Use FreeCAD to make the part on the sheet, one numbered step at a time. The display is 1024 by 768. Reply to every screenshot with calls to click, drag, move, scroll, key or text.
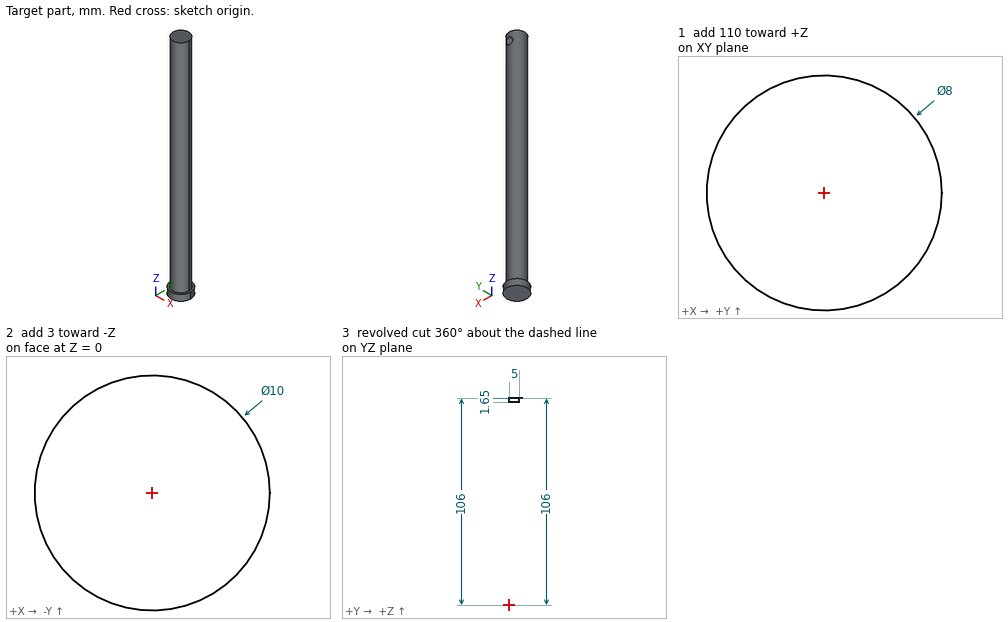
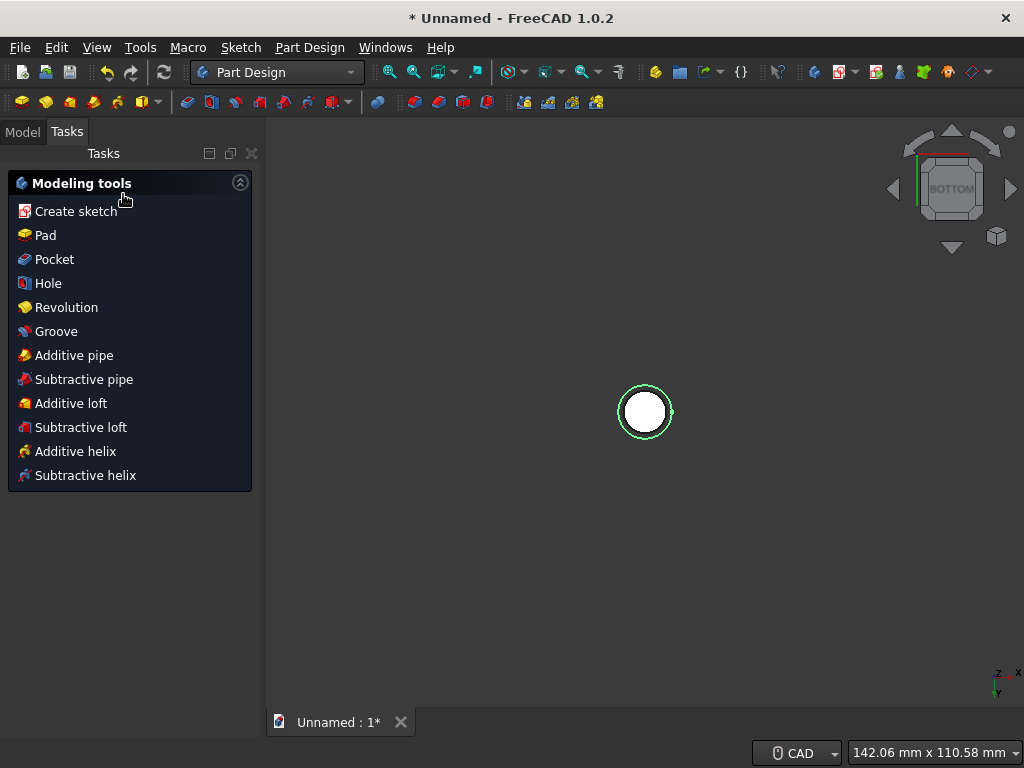
click(22, 102)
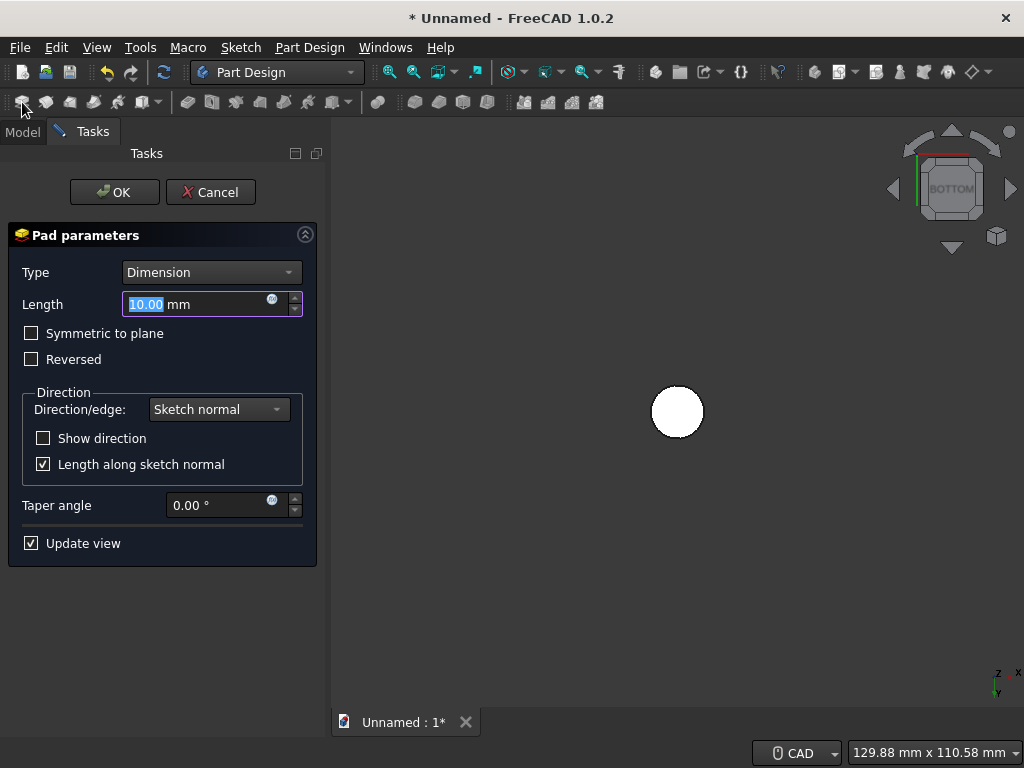
text(3)
key(Tab)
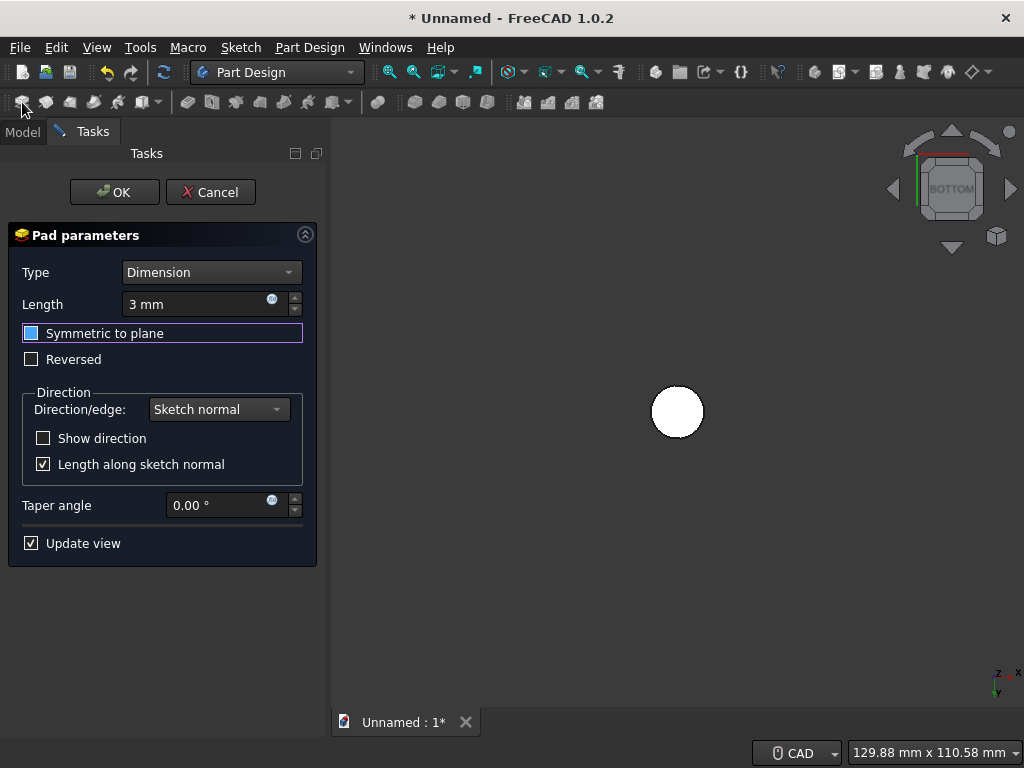
click(115, 192)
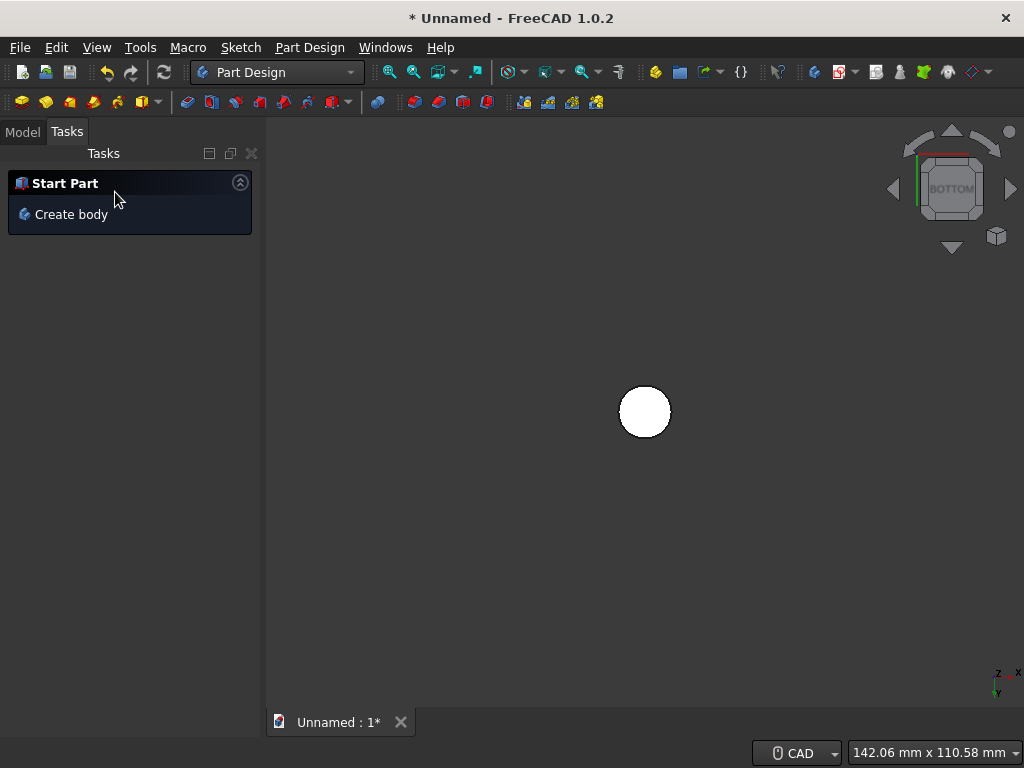
click(390, 72)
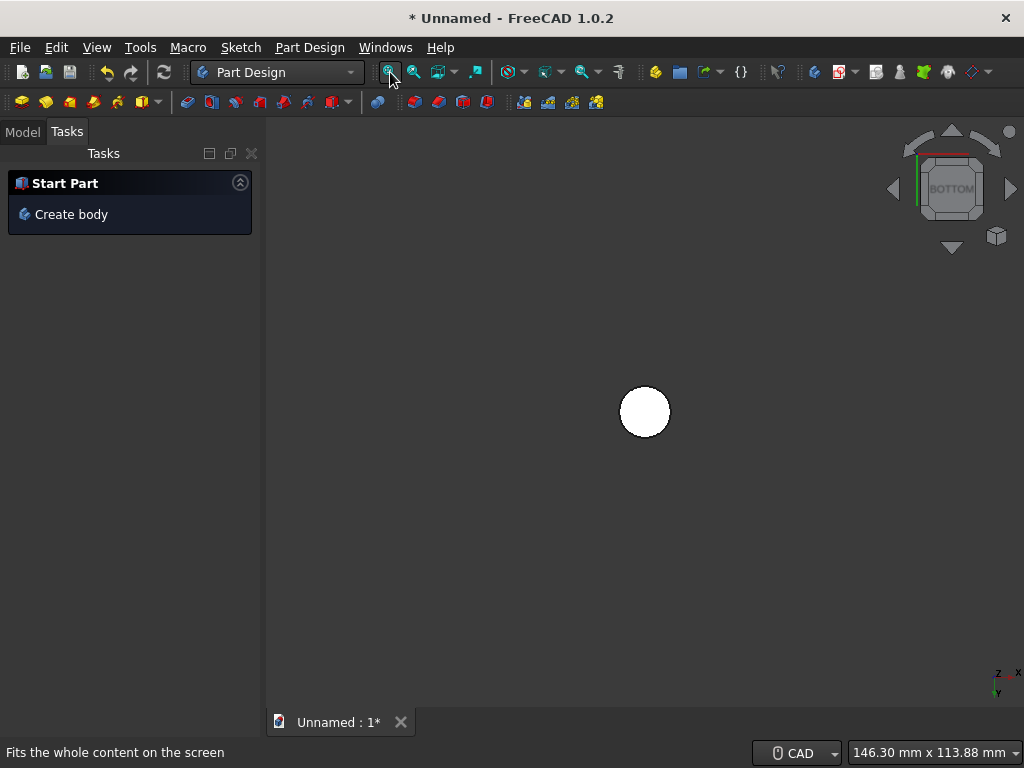
click(840, 72)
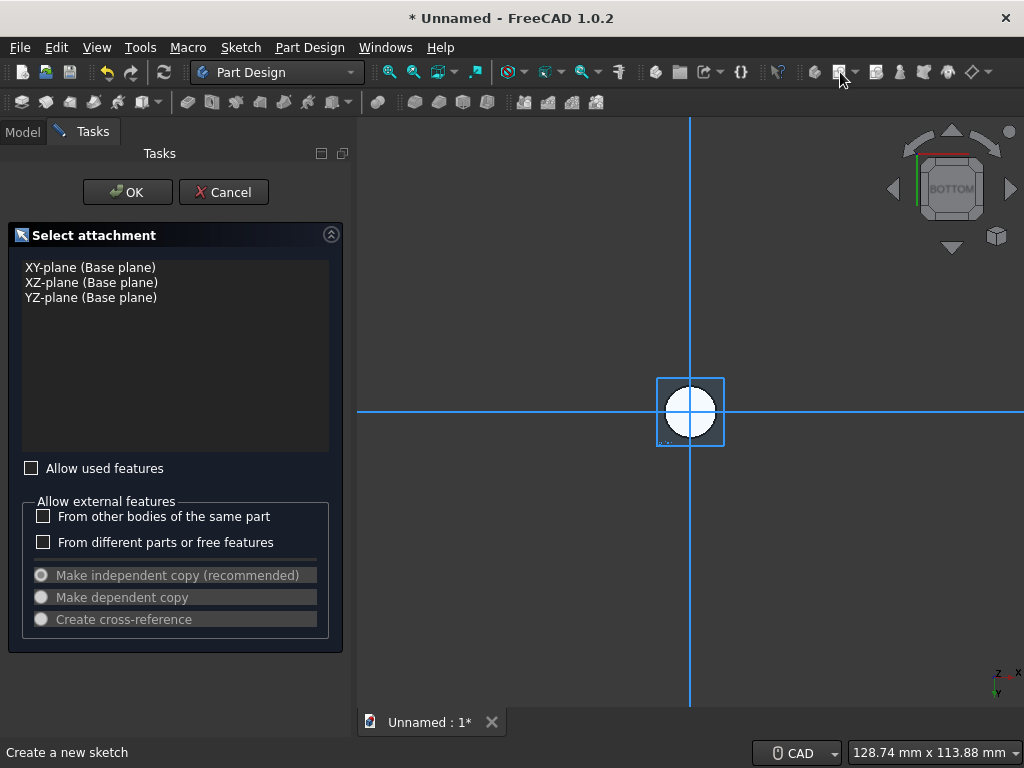
click(82, 298)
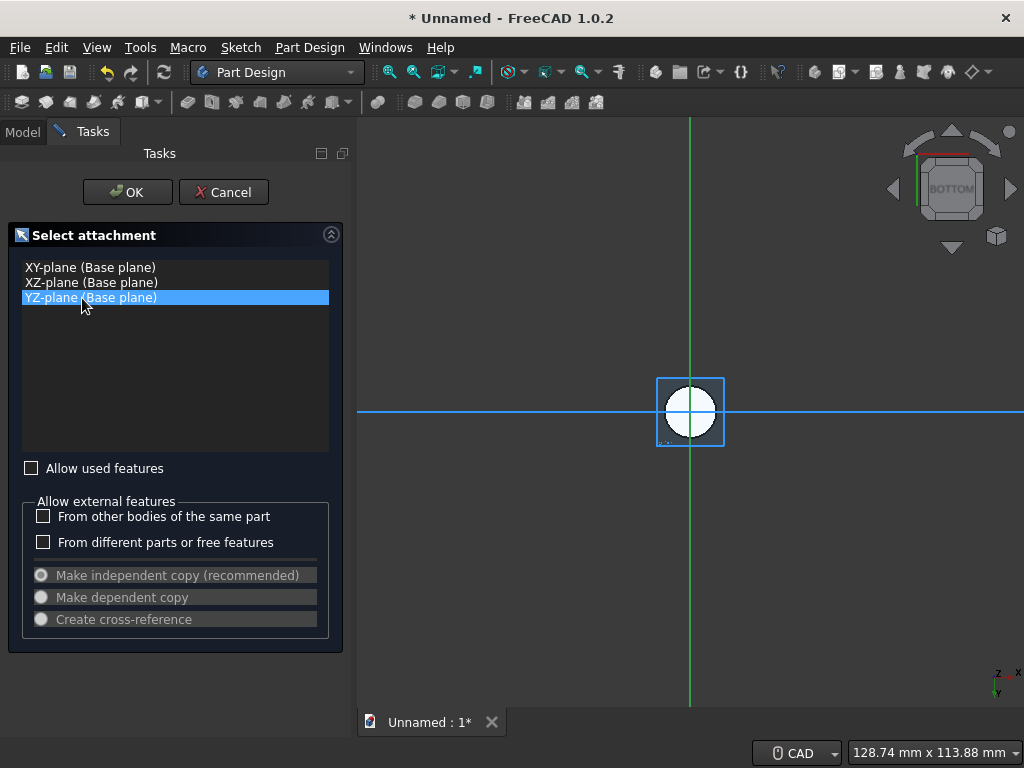
click(128, 192)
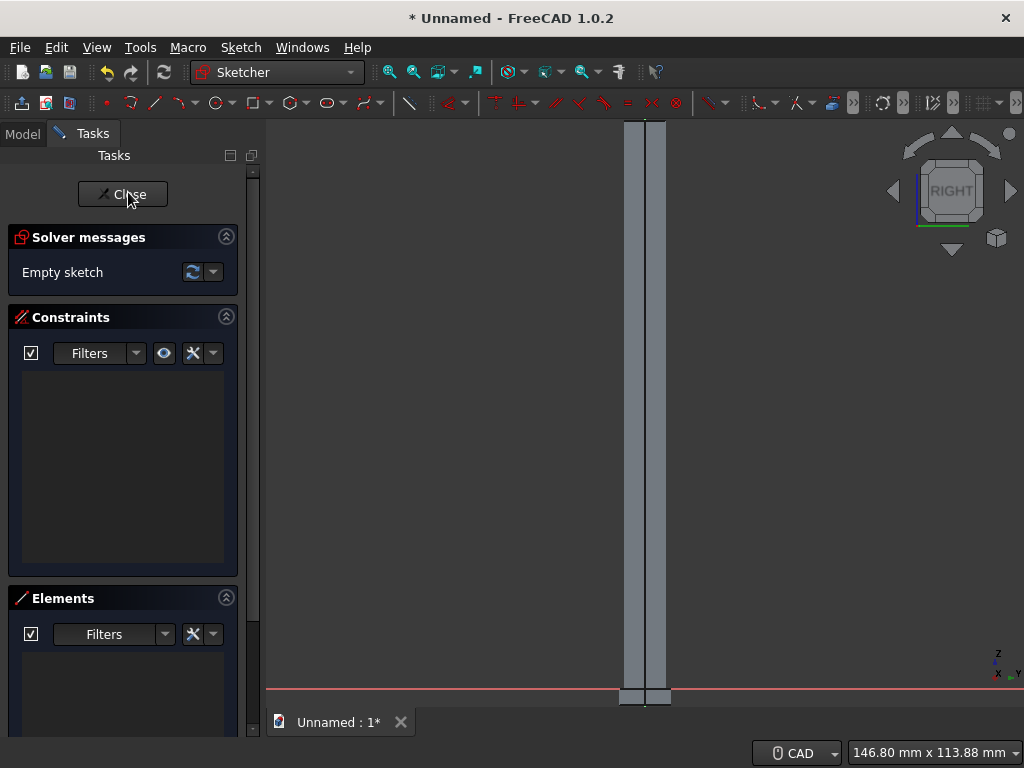
click(70, 104)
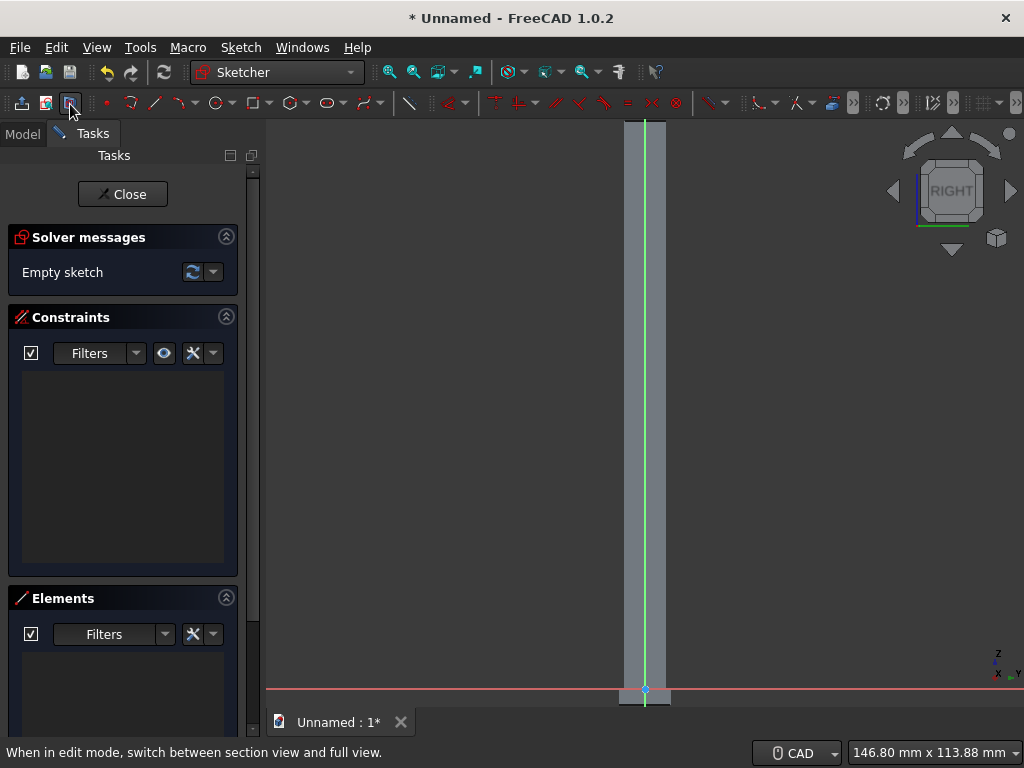
scroll(576, 413, down, 5)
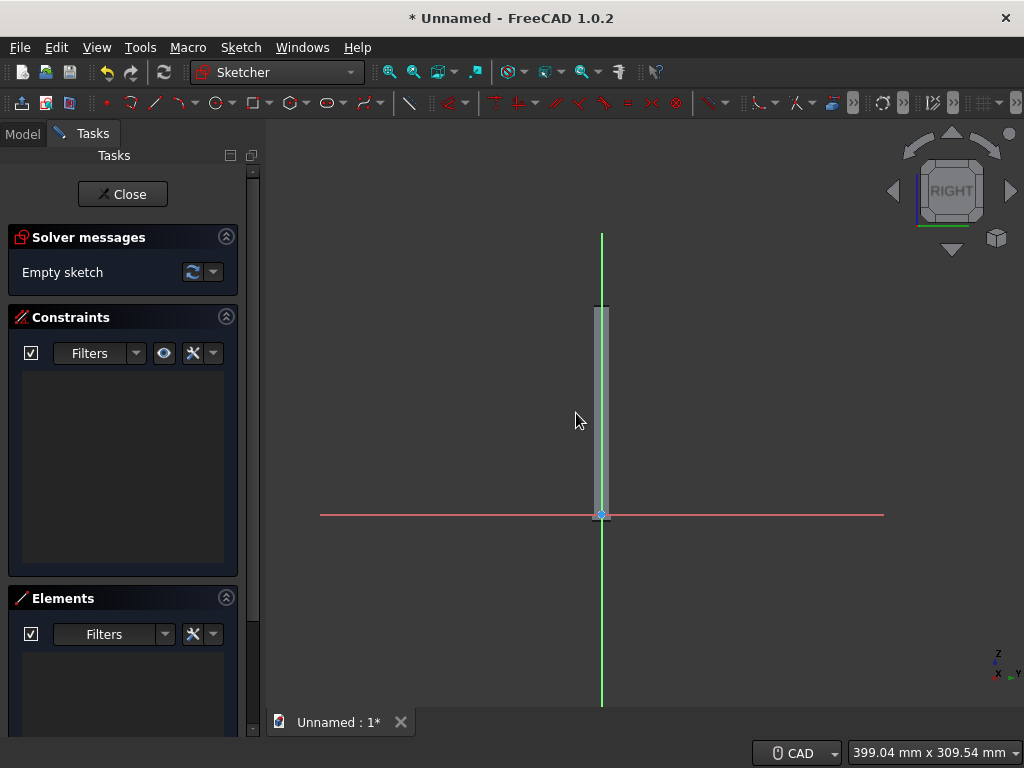
scroll(610, 310, up, 15)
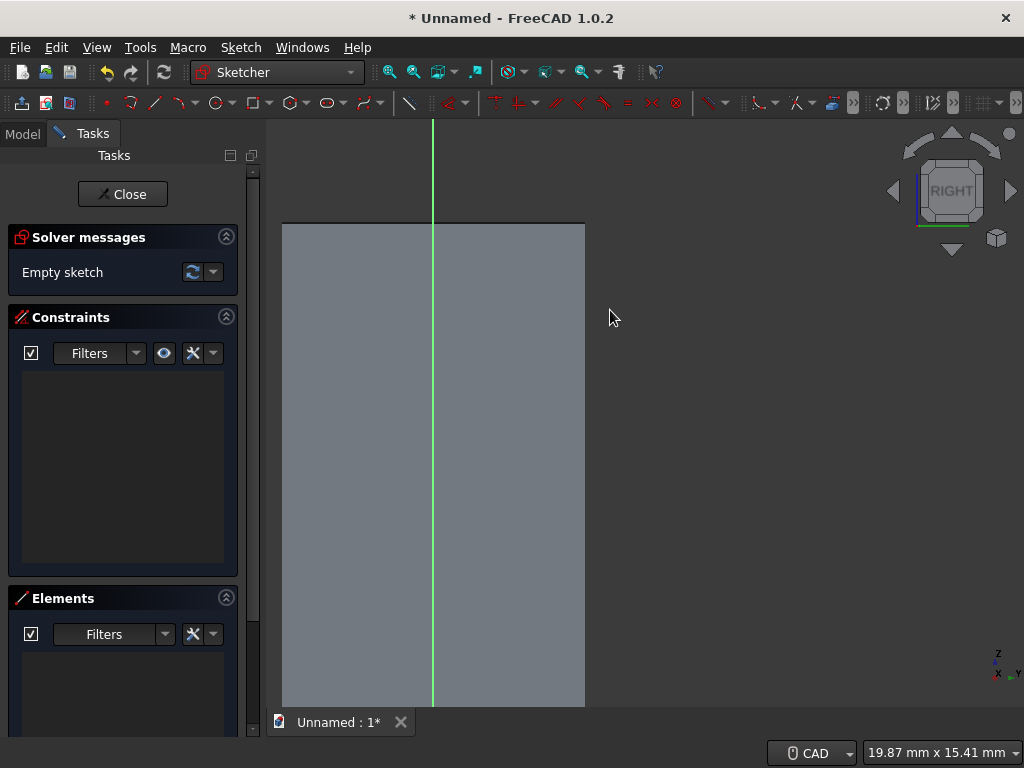
scroll(548, 396, up, 2)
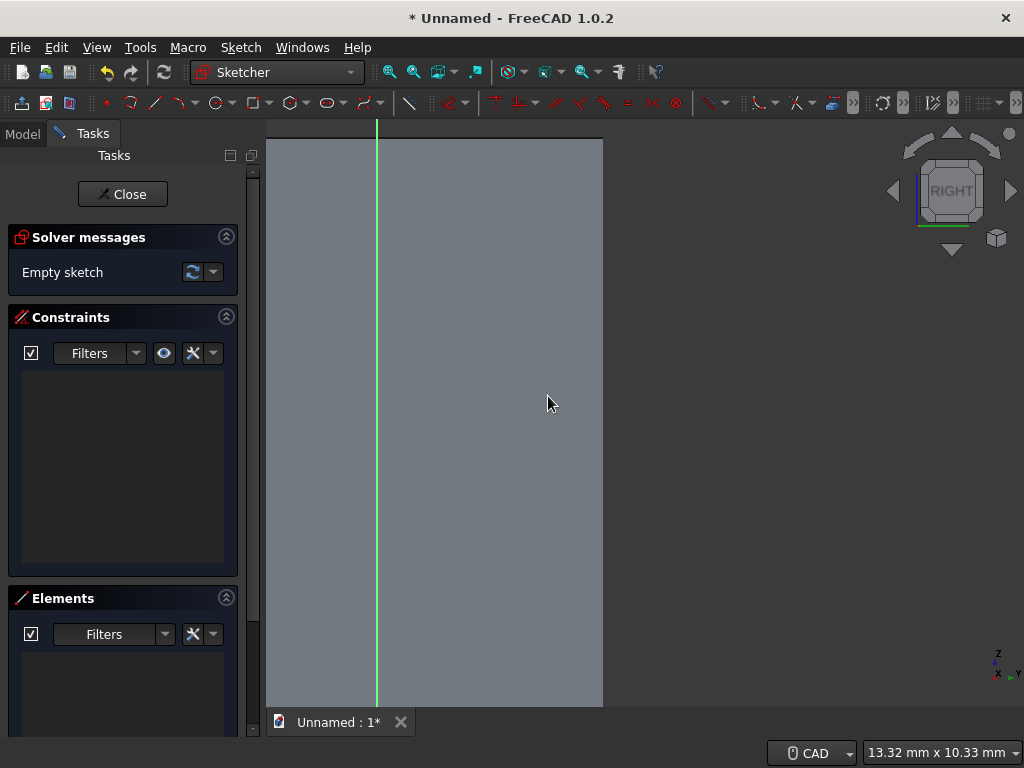
click(254, 104)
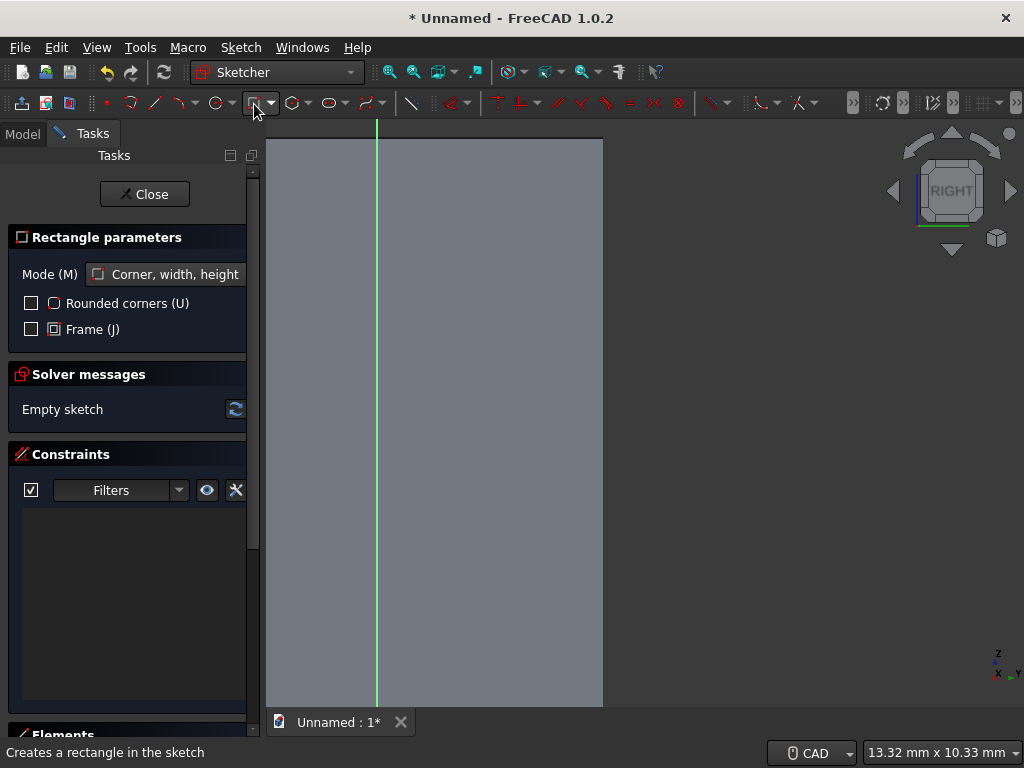
click(377, 366)
click(662, 460)